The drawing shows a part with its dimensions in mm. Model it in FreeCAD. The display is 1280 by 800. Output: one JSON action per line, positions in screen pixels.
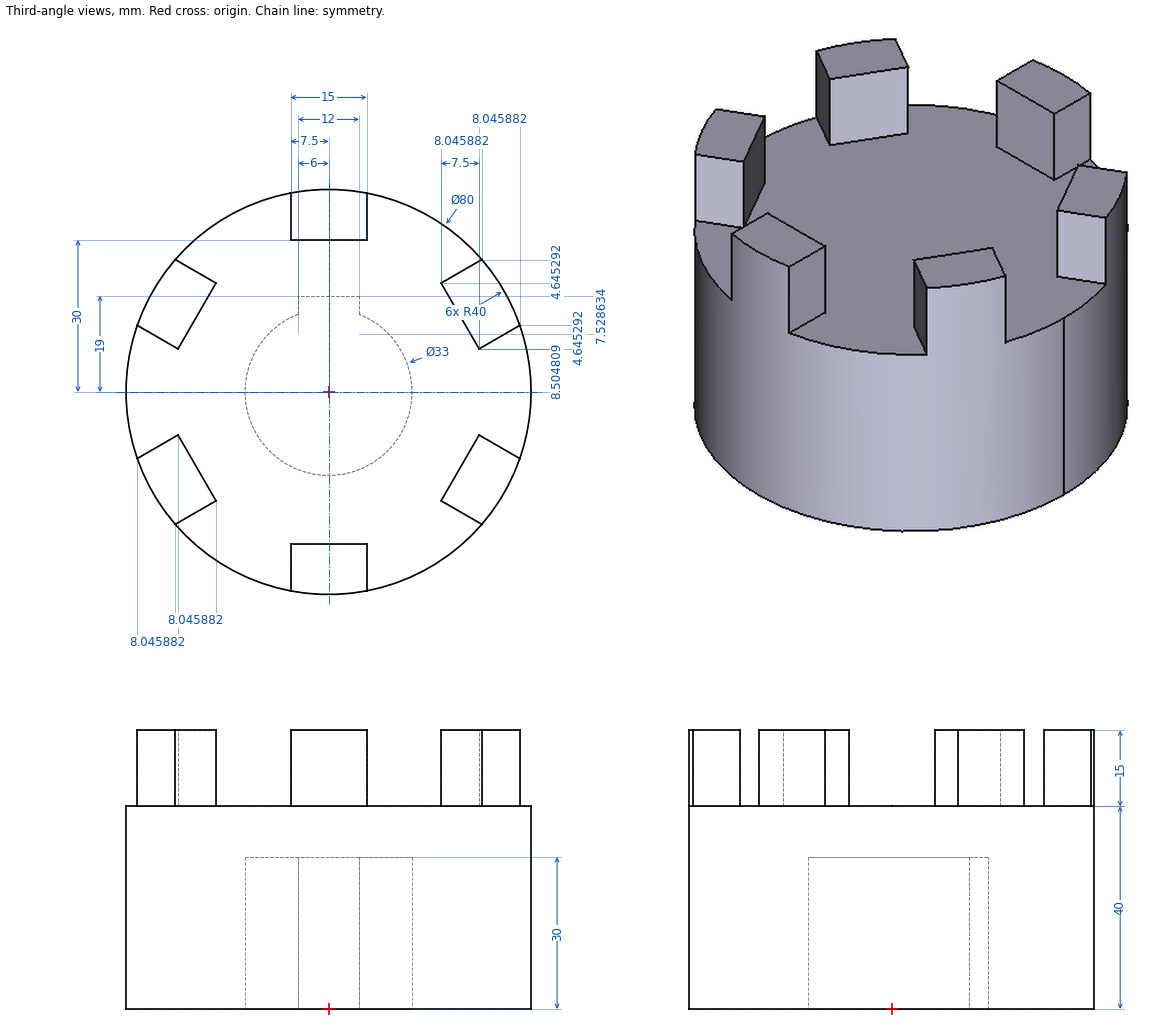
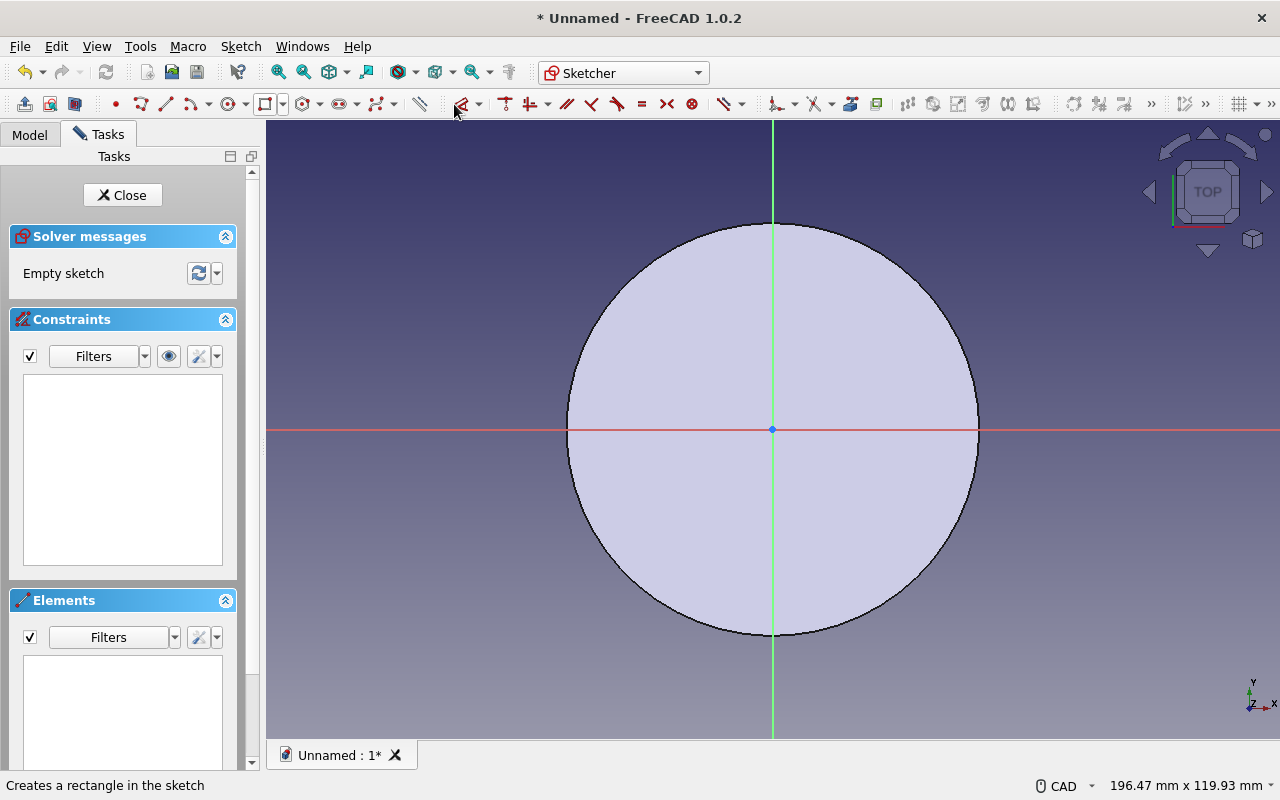
{"action": "left_click", "coordinate": [929, 295]}
{"action": "left_click", "coordinate": [888, 319]}
{"action": "left_click", "coordinate": [926, 386]}
{"action": "left_click", "coordinate": [968, 362]}
{"action": "right_click", "coordinate": [968, 362]}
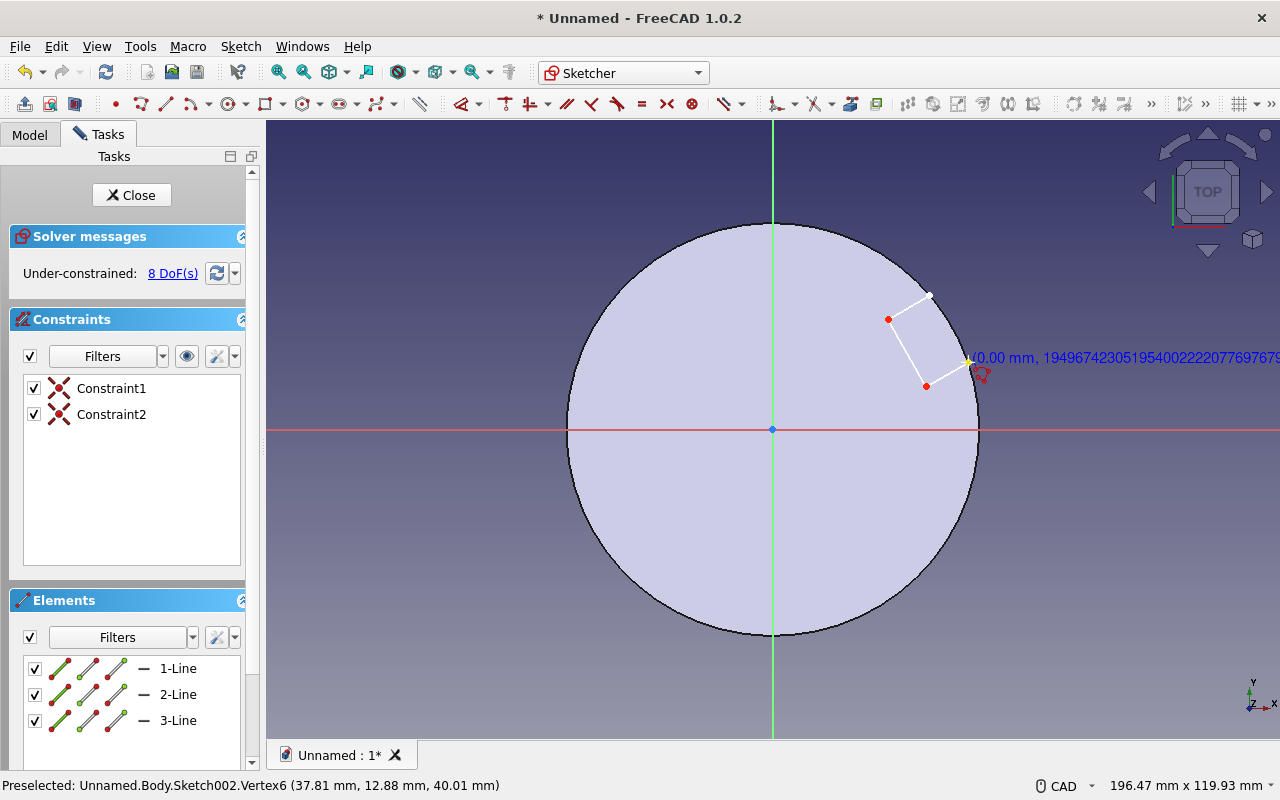
{"action": "key", "text": "g 3 a"}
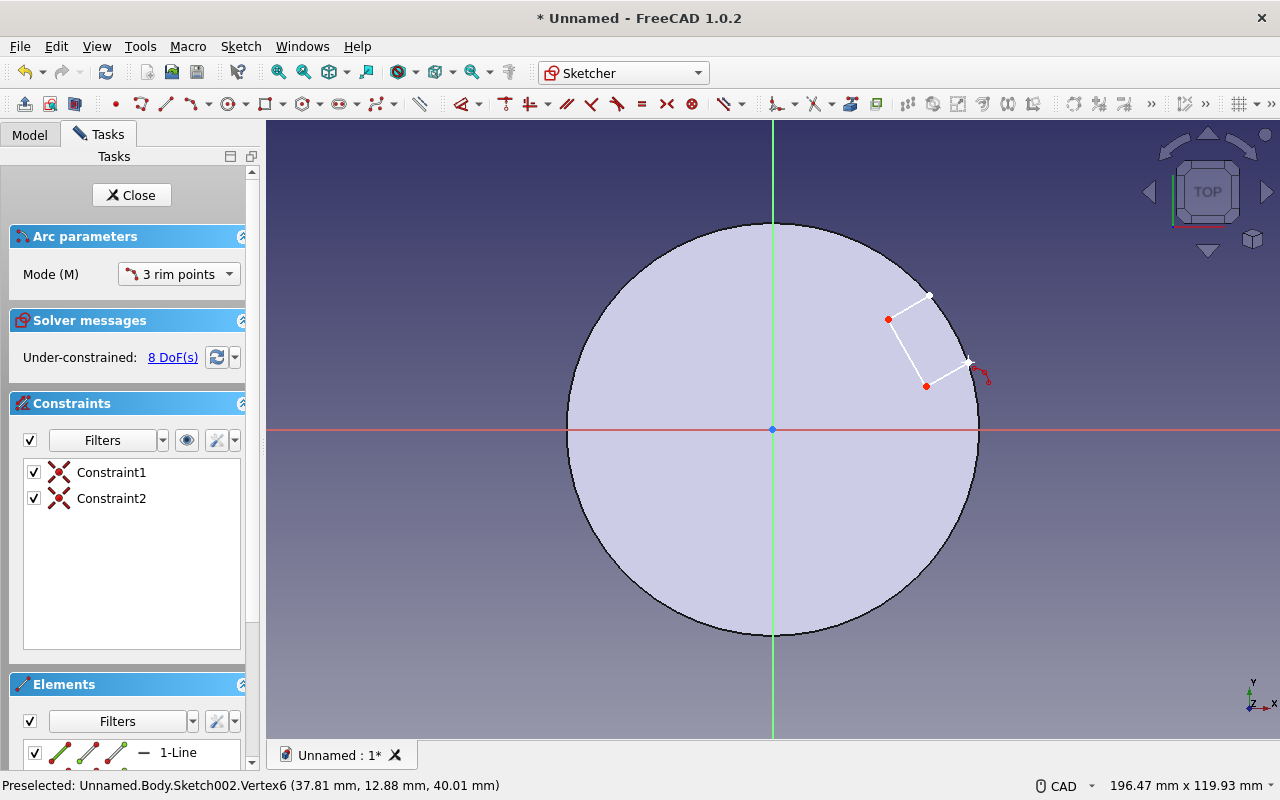
{"action": "left_click", "coordinate": [968, 363]}
{"action": "left_click", "coordinate": [929, 296]}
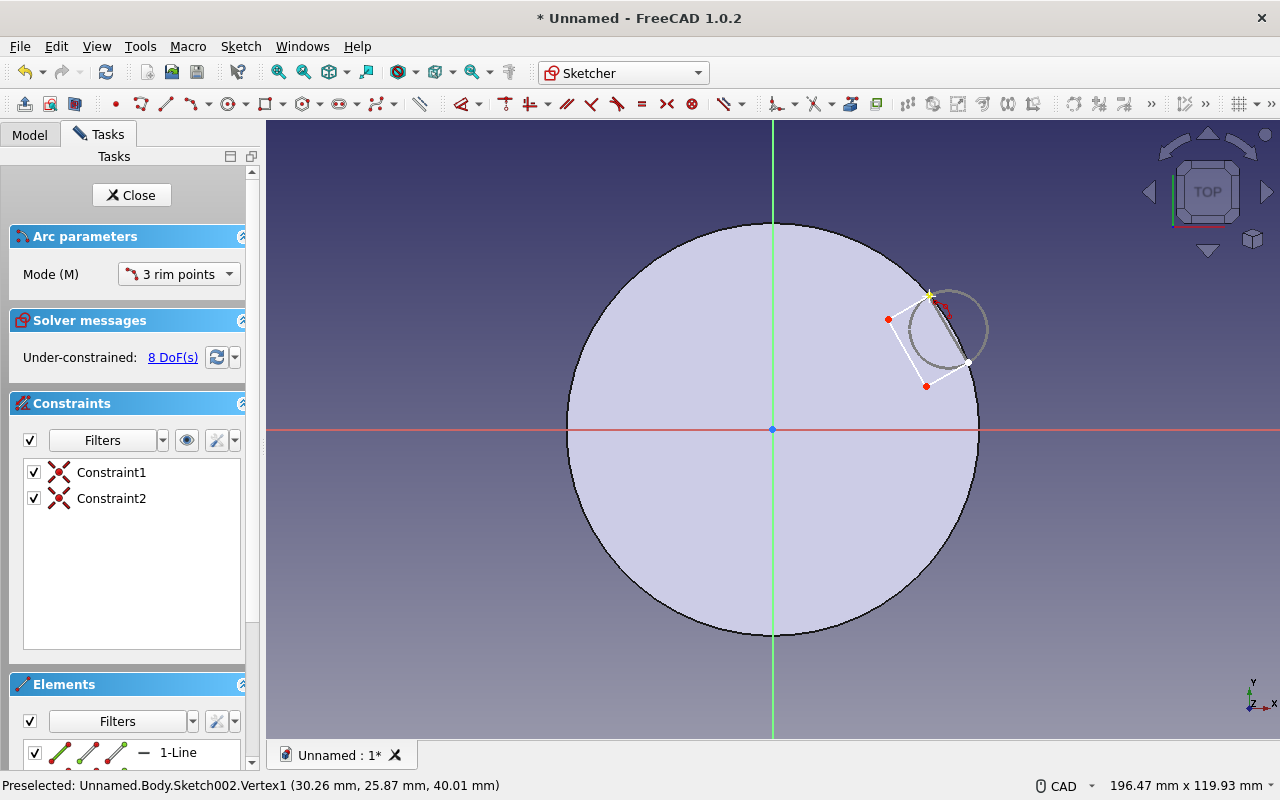
{"action": "scroll", "coordinate": [952, 326], "scroll_direction": "up", "scroll_amount": 8}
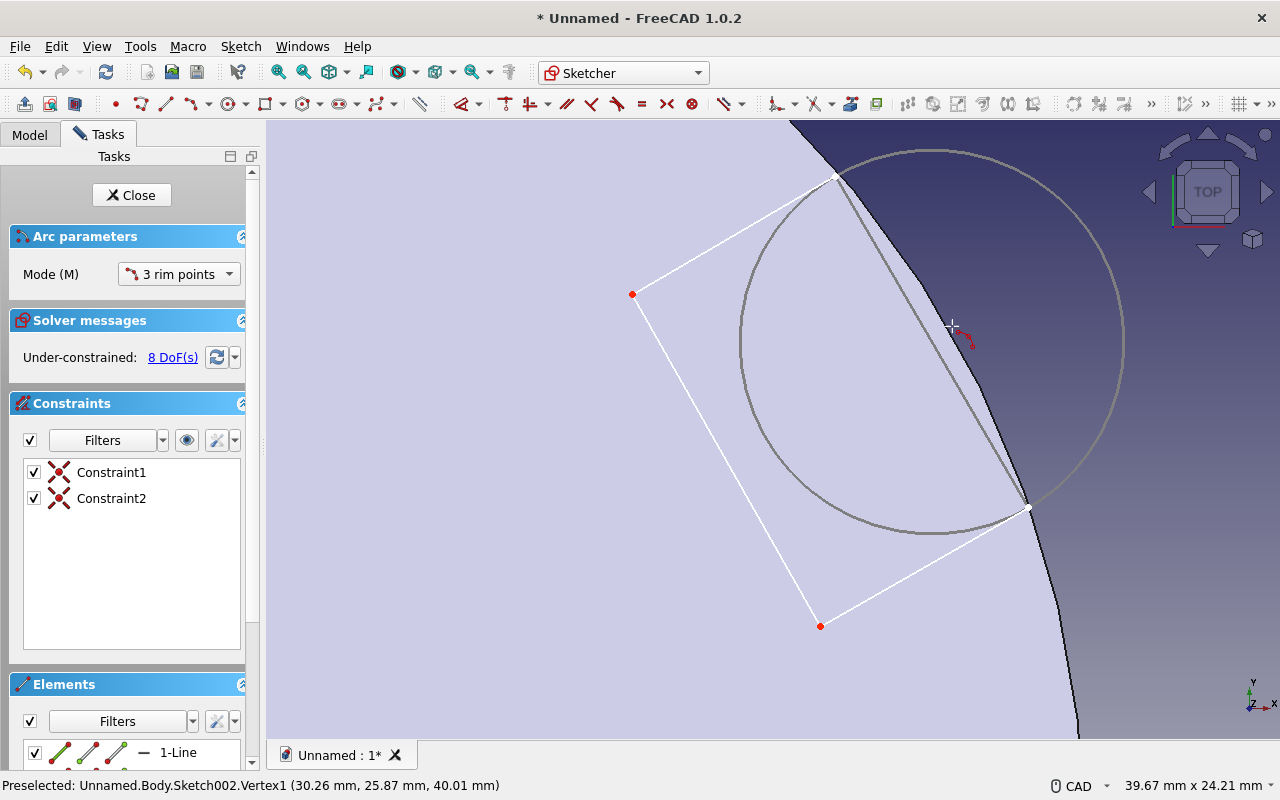
{"action": "left_click", "coordinate": [947, 326]}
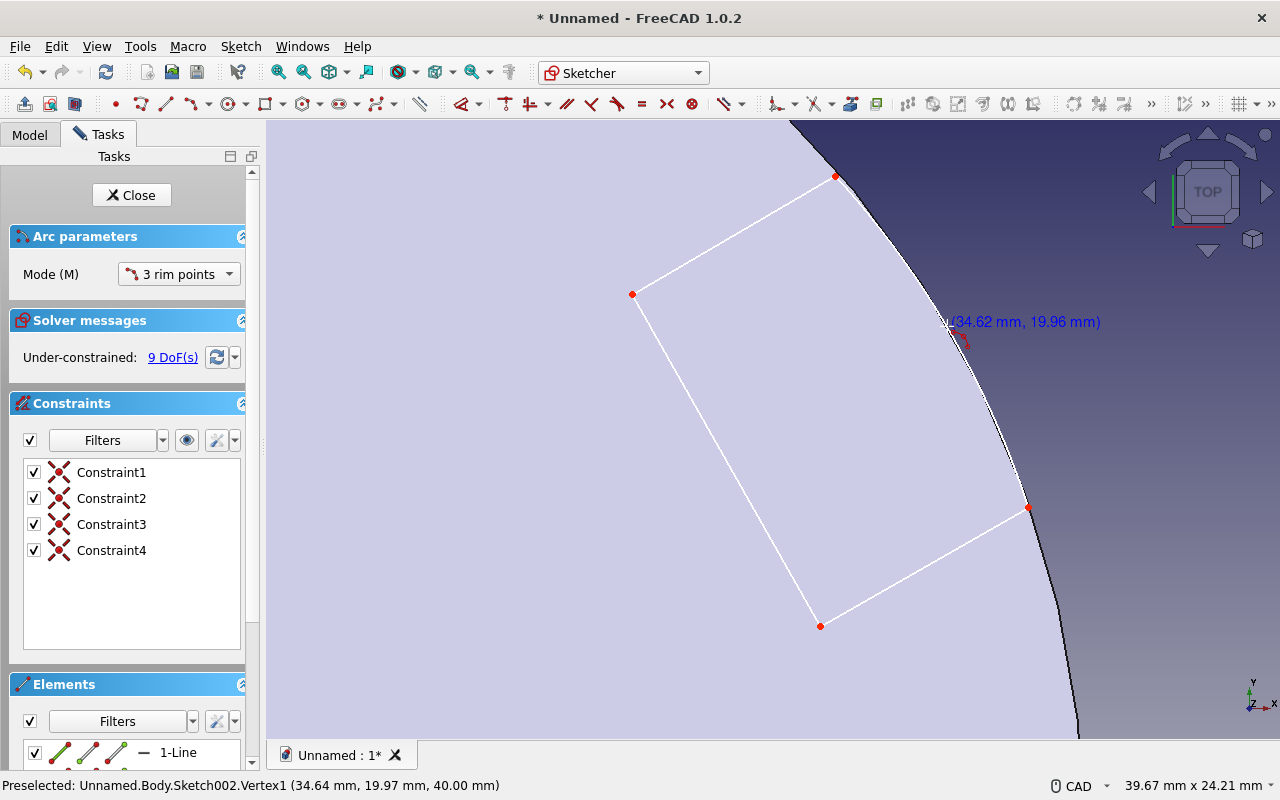
{"action": "key", "text": "g m"}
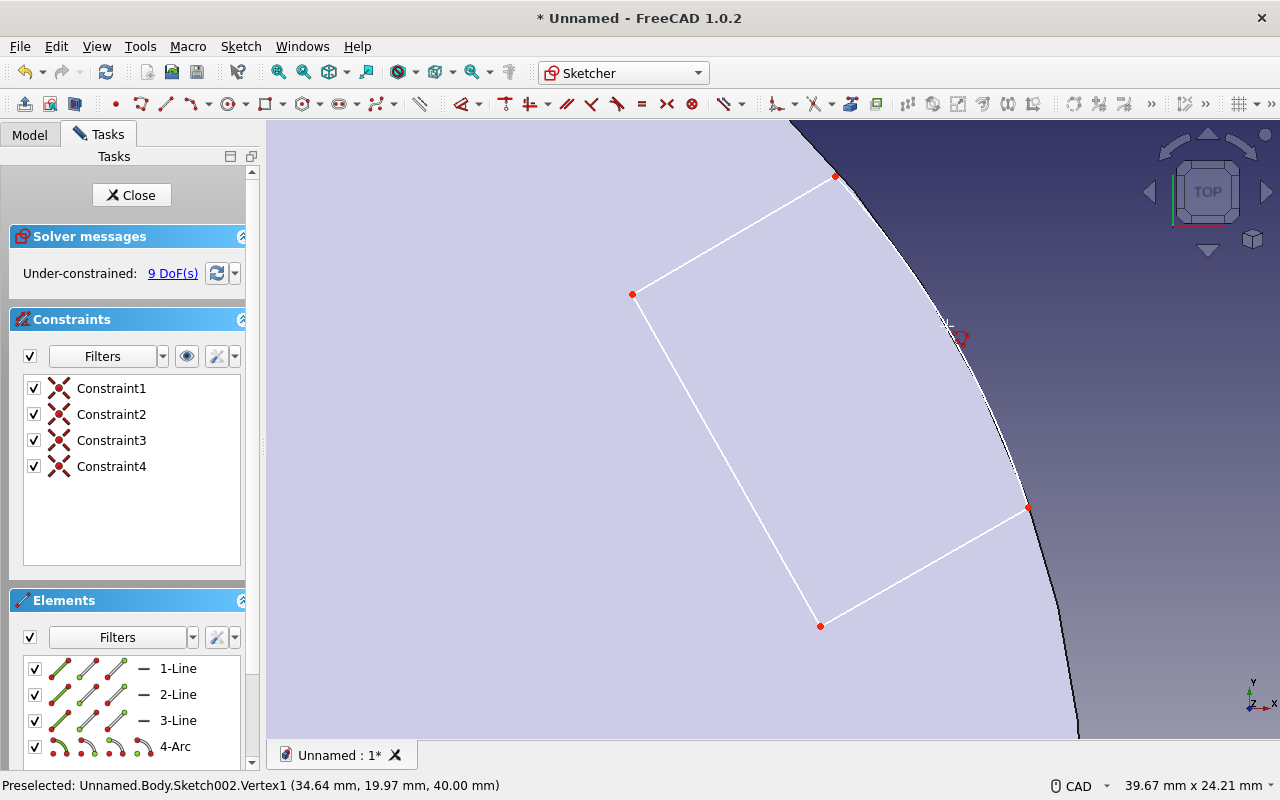
{"action": "scroll", "coordinate": [867, 326], "scroll_direction": "down", "scroll_amount": 8}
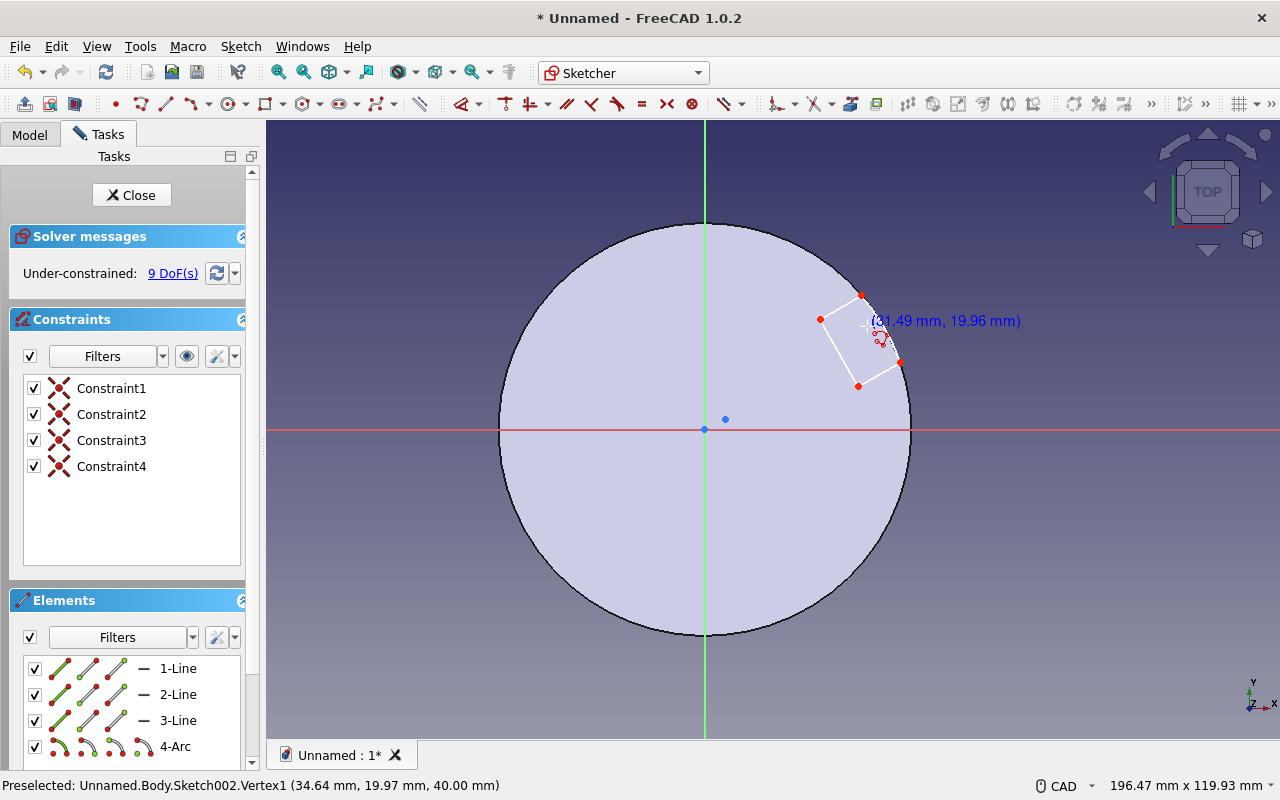
{"action": "left_click", "coordinate": [666, 227]}
{"action": "left_click", "coordinate": [666, 275]}
{"action": "left_click", "coordinate": [744, 275]}
{"action": "left_click", "coordinate": [744, 227]}
{"action": "right_click", "coordinate": [744, 227]}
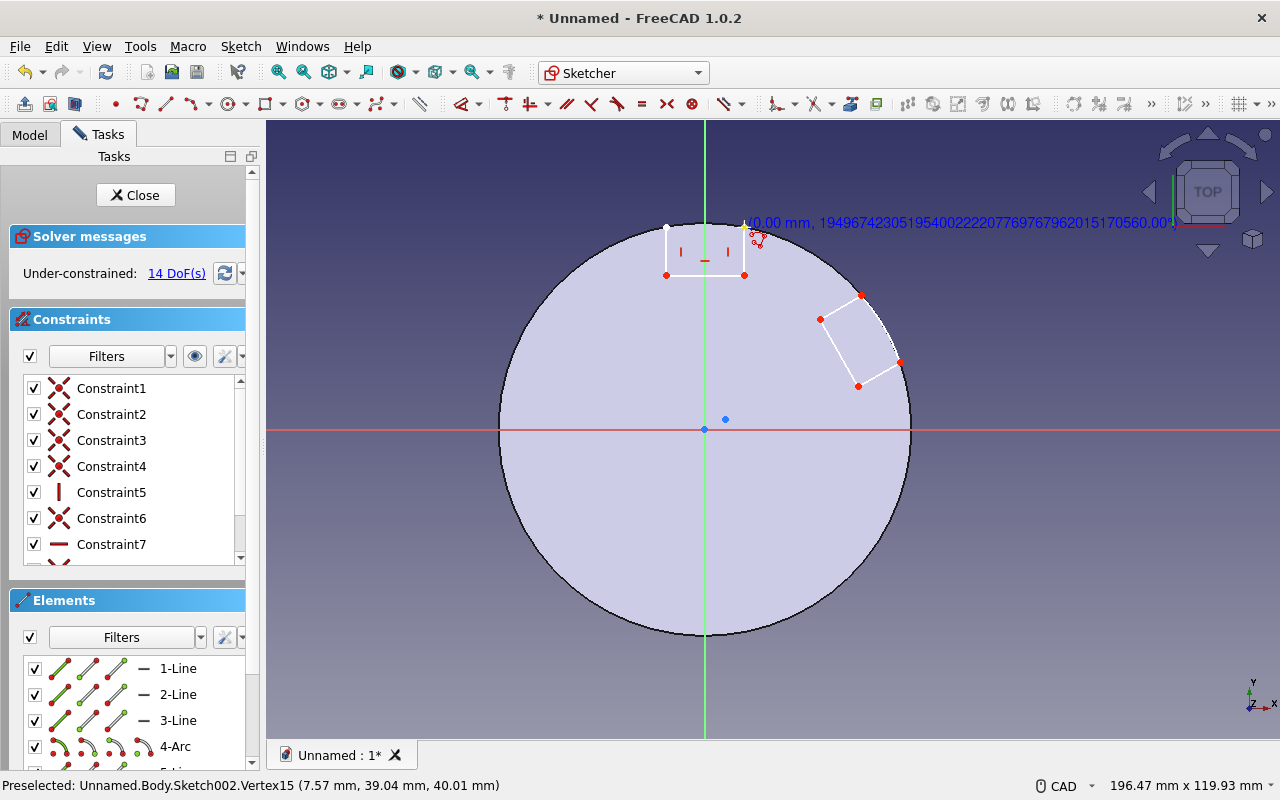
{"action": "left_click", "coordinate": [190, 104]}